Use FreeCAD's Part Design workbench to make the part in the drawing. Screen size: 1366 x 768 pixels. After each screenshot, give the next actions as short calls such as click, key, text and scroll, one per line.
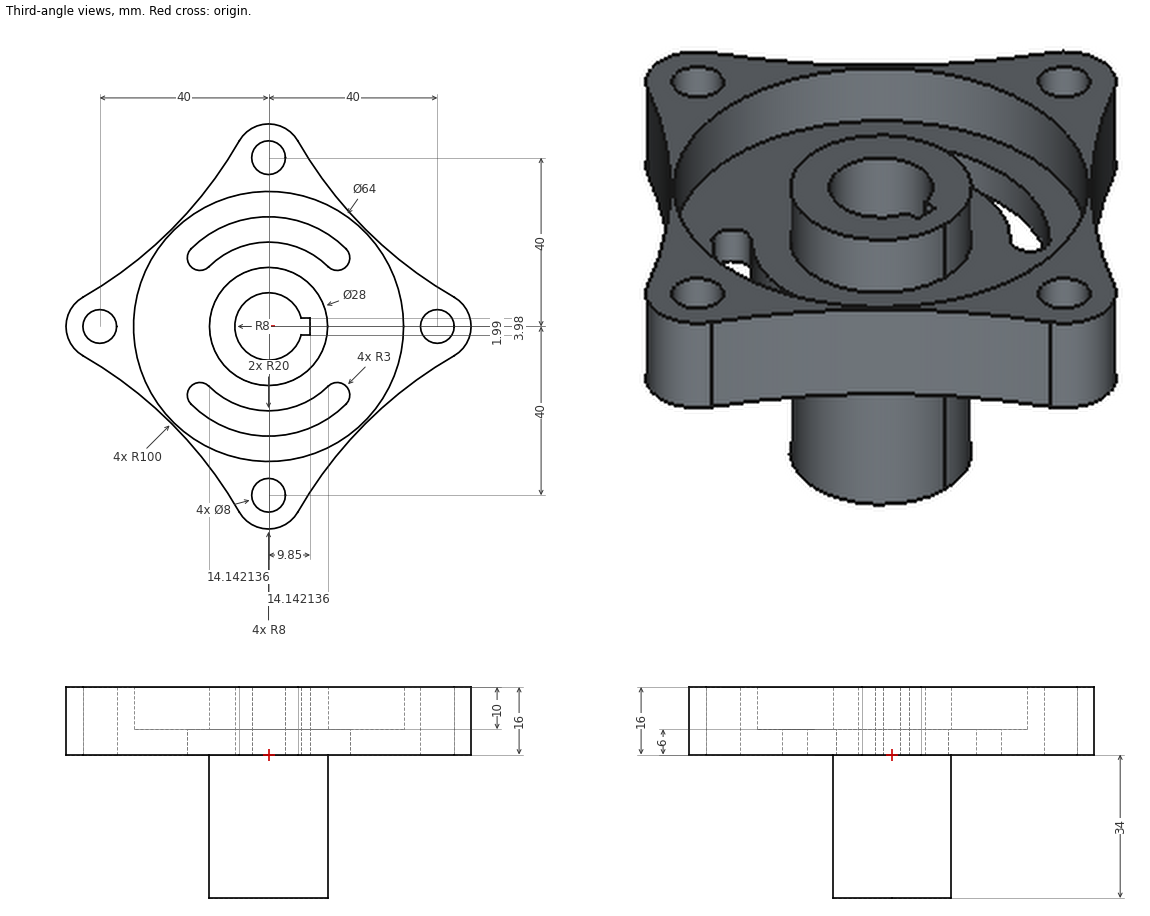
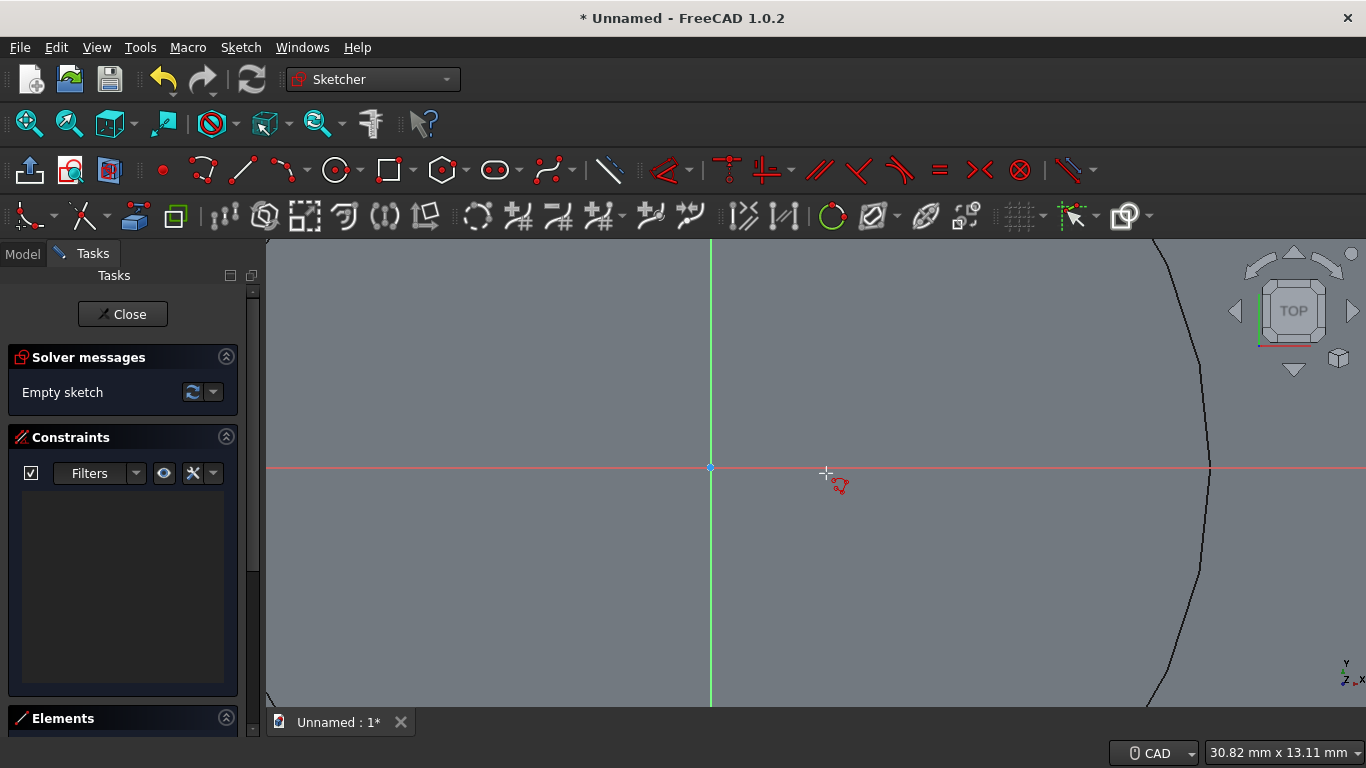
click(987, 539)
click(1062, 539)
click(1062, 397)
click(987, 397)
right_click(987, 397)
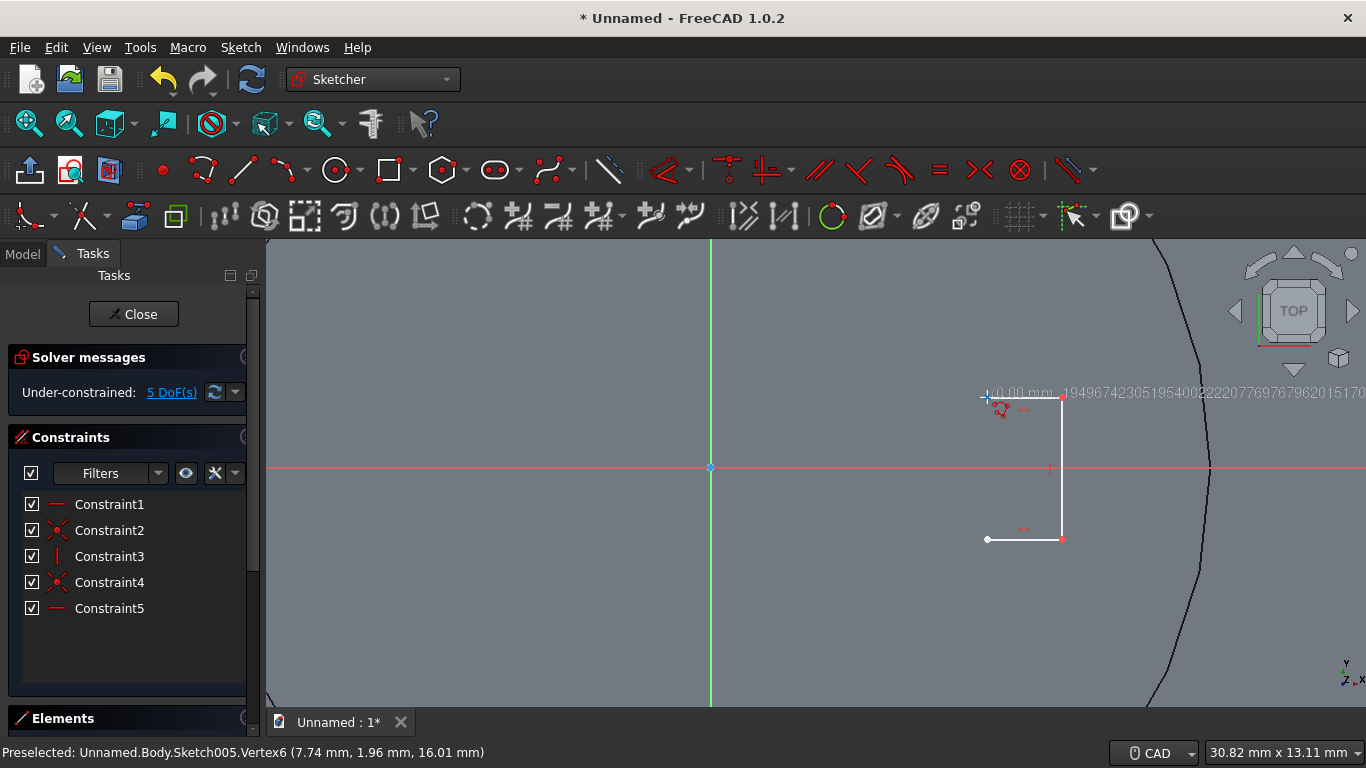
click(284, 170)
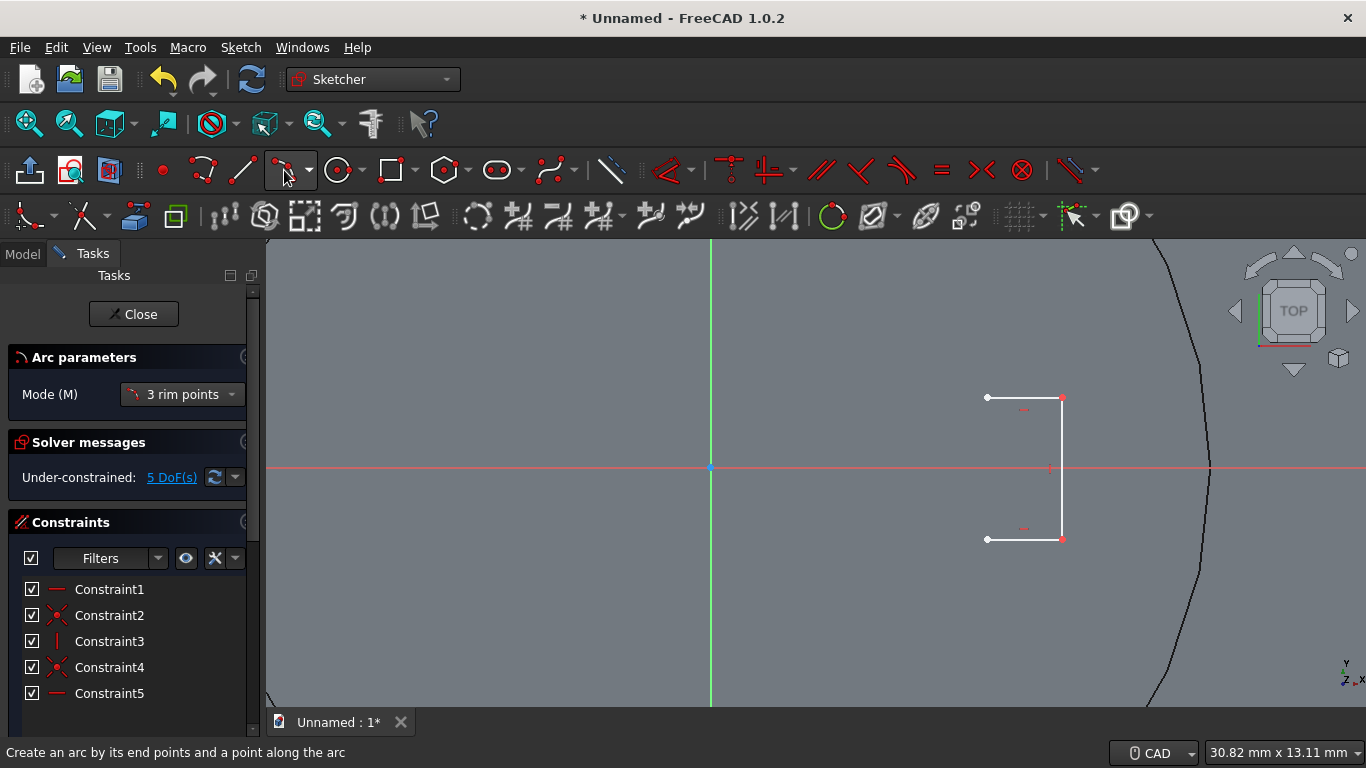
click(987, 398)
click(987, 540)
click(472, 312)
key(Escape)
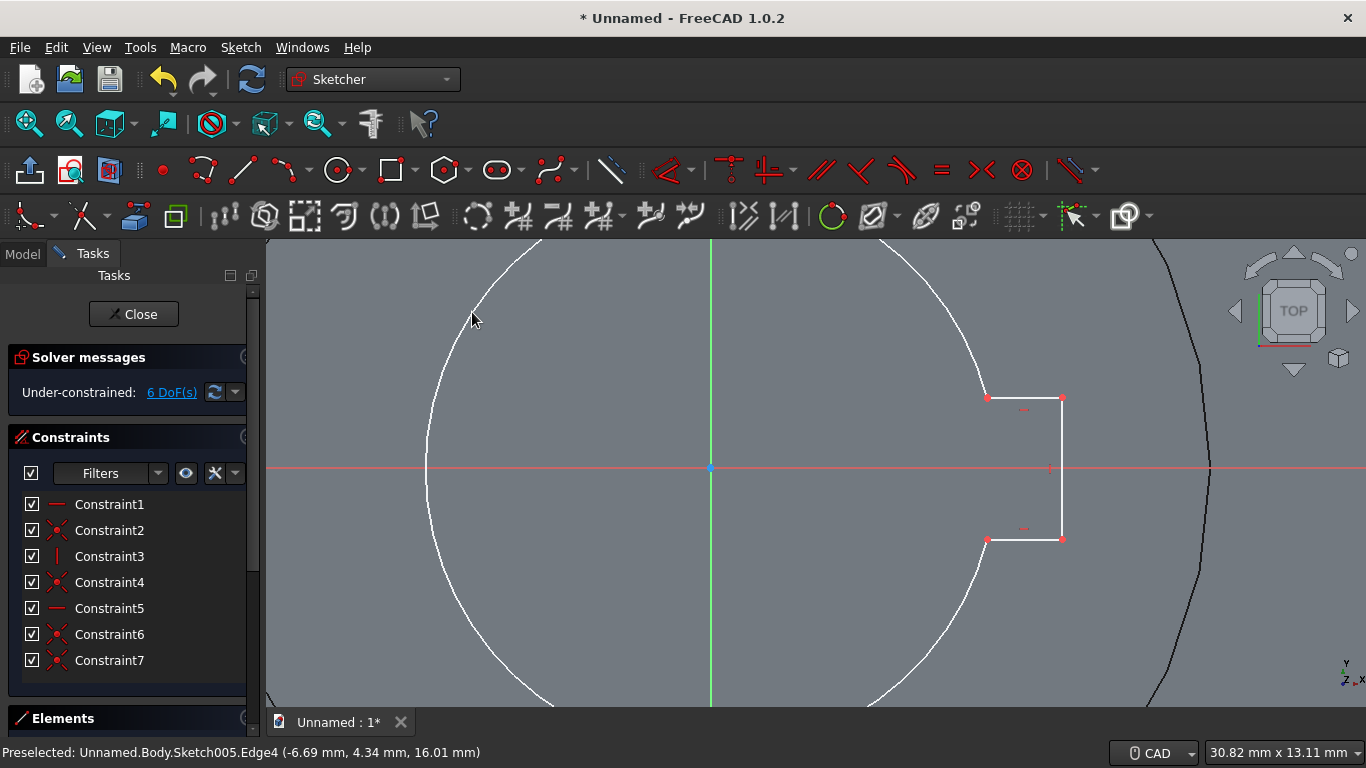
drag(701, 458, 721, 479)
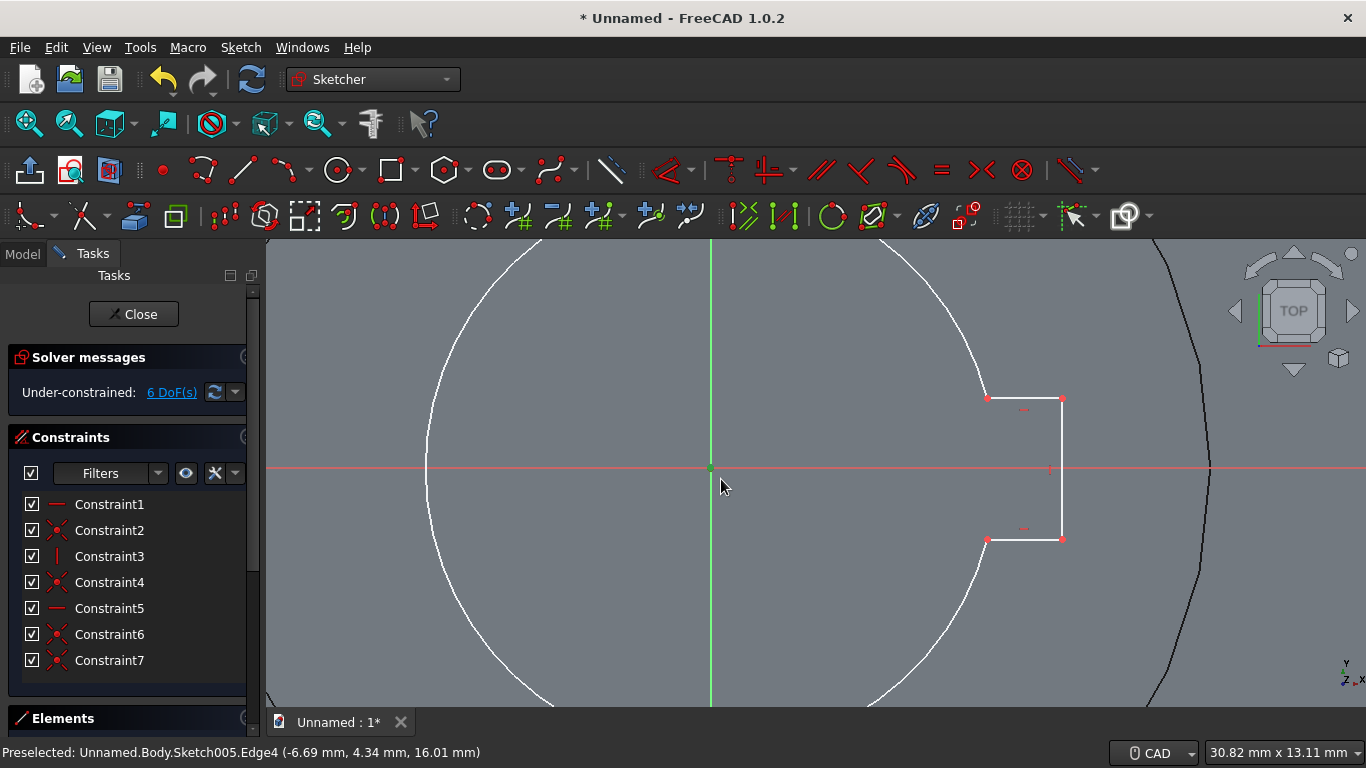
click(730, 170)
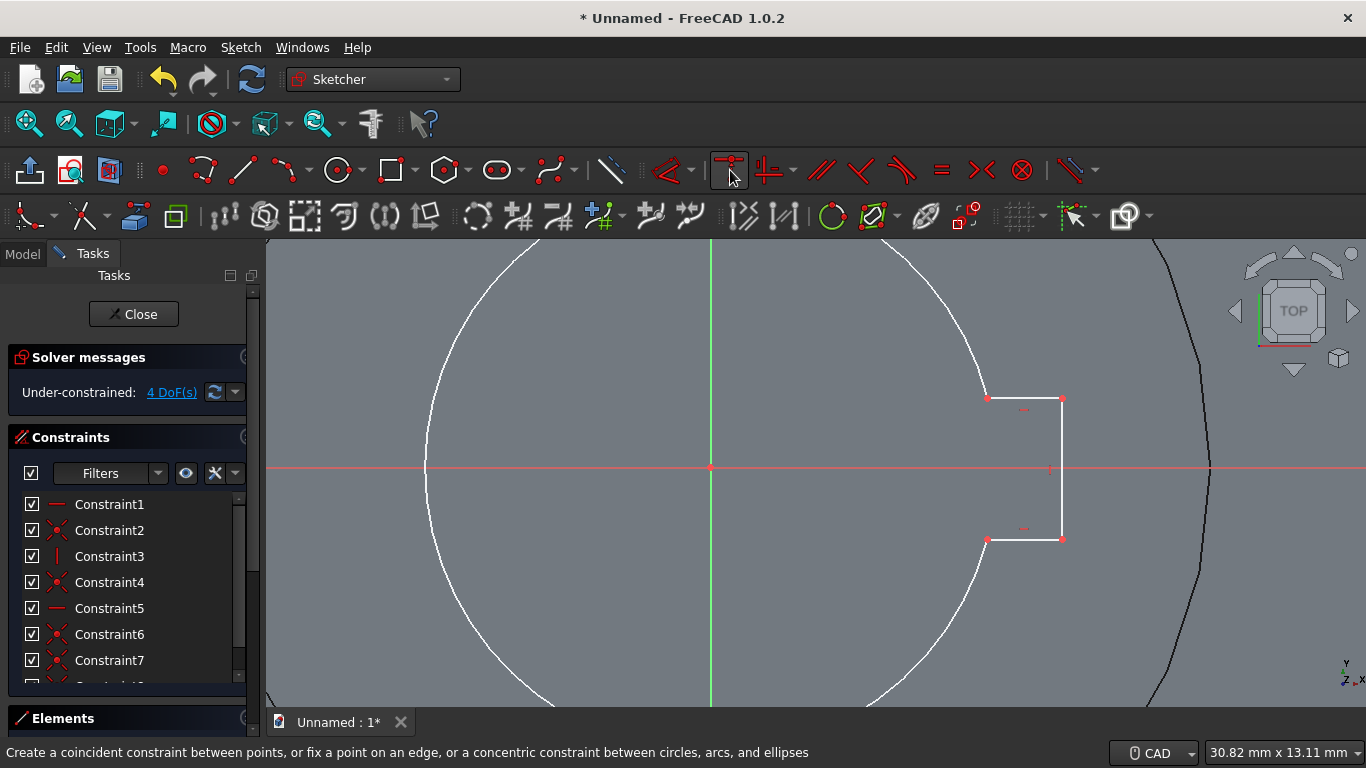
click(666, 170)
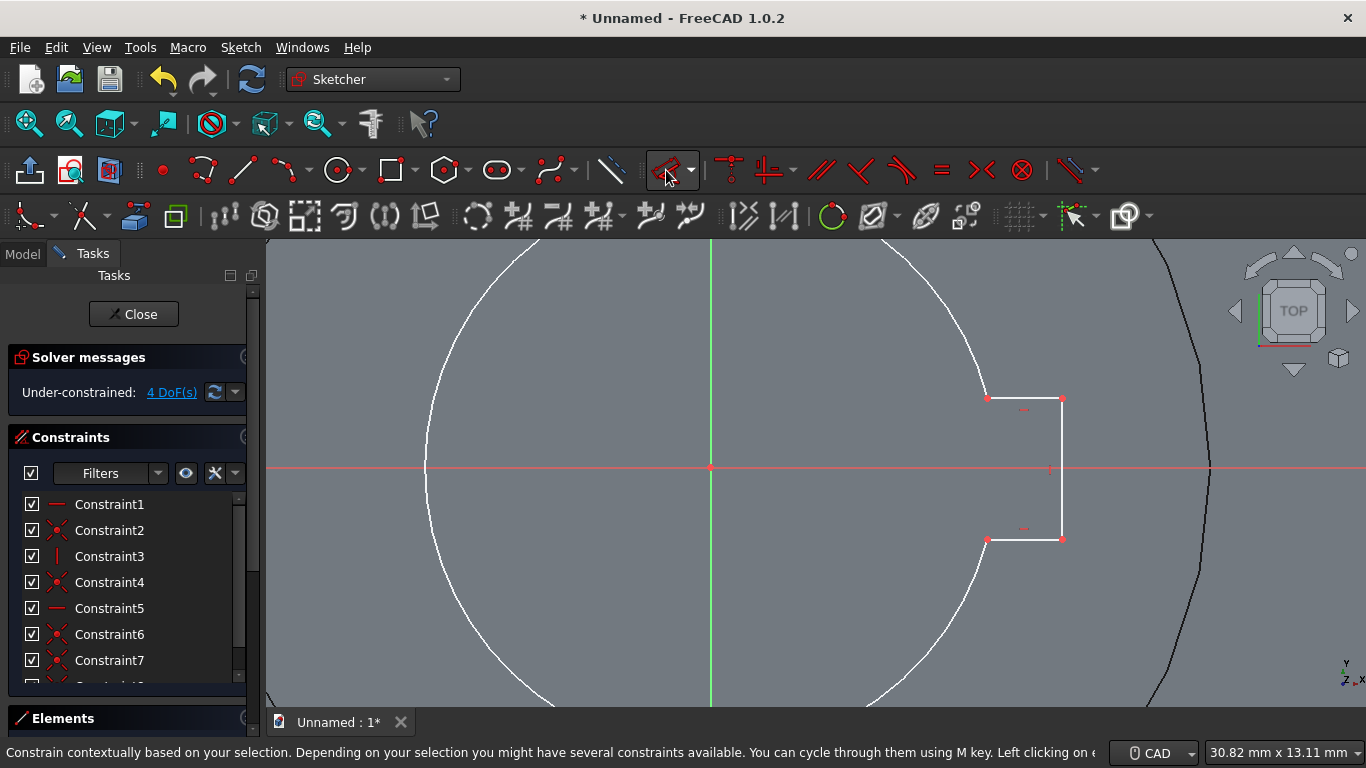
click(425, 467)
click(432, 315)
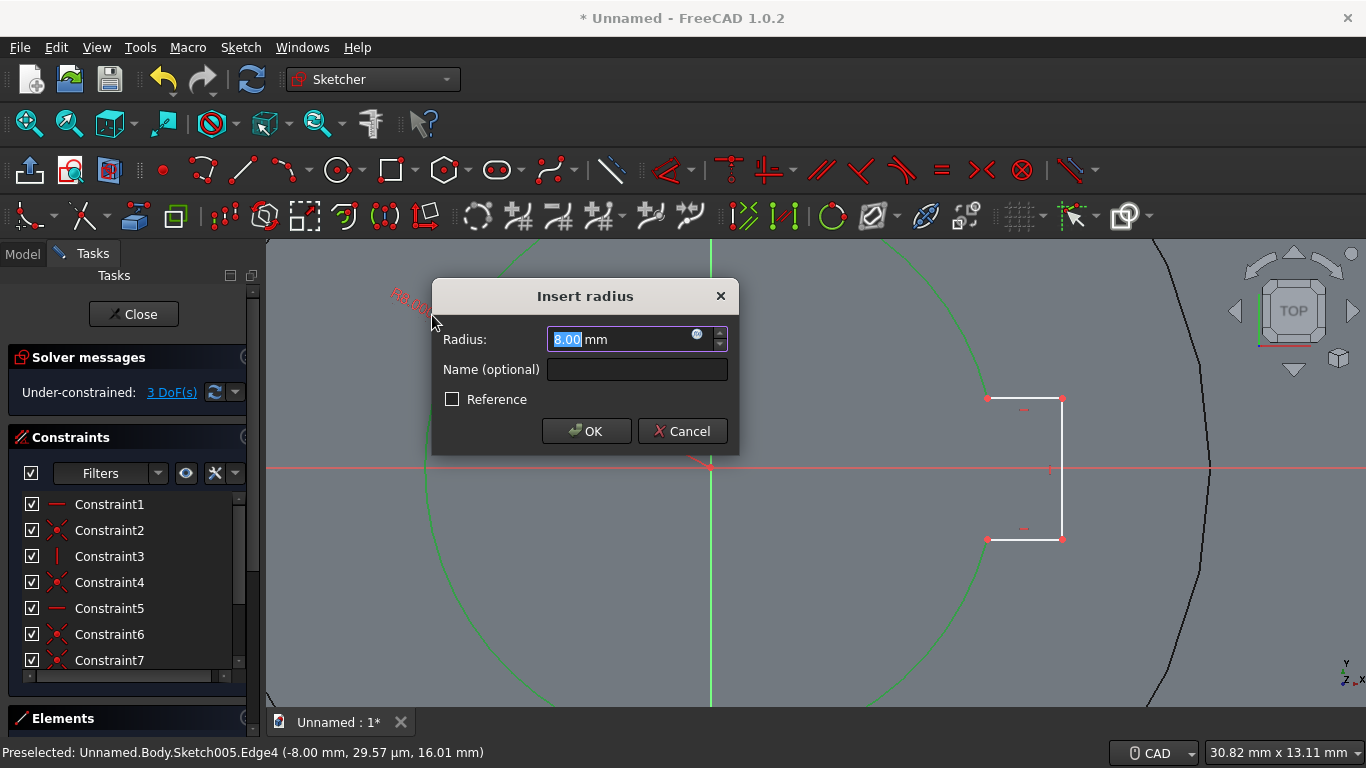
text(8)
key(Return)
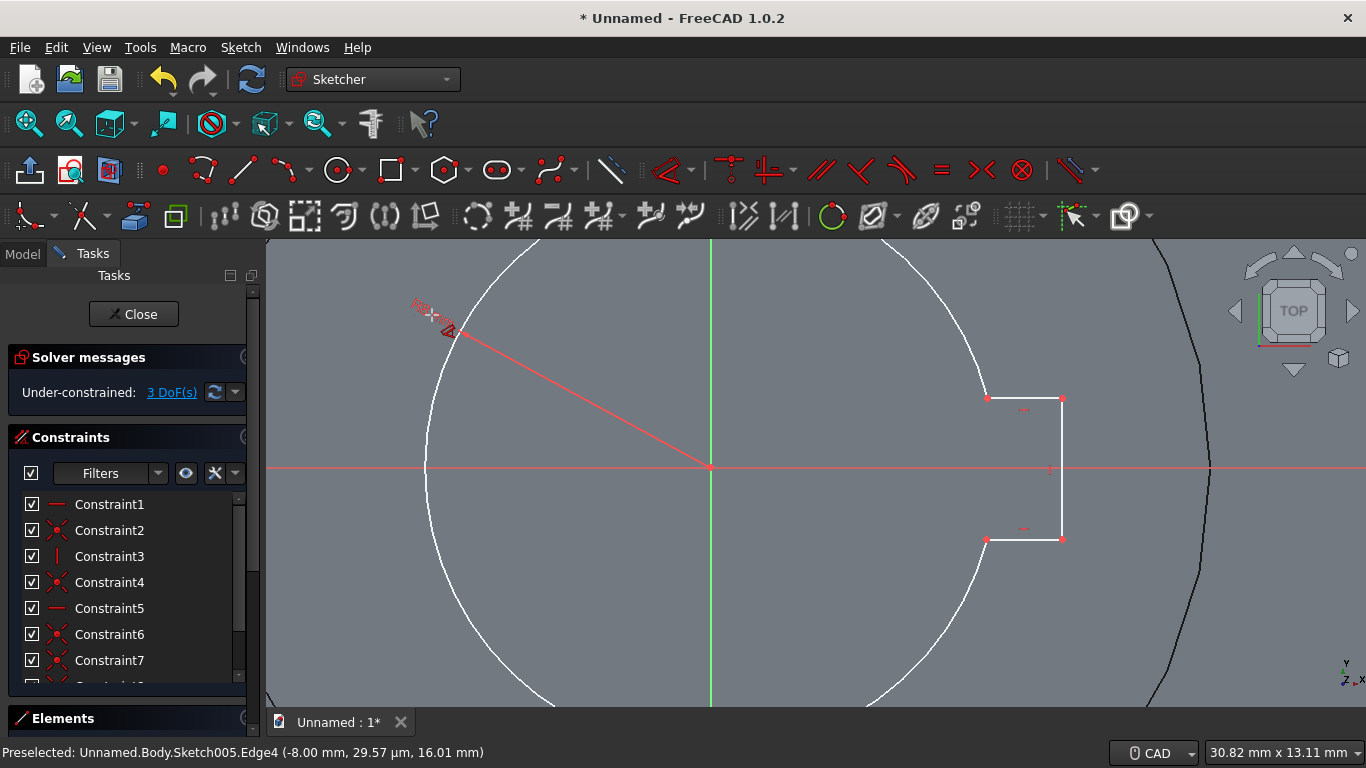
click(1062, 497)
click(1096, 436)